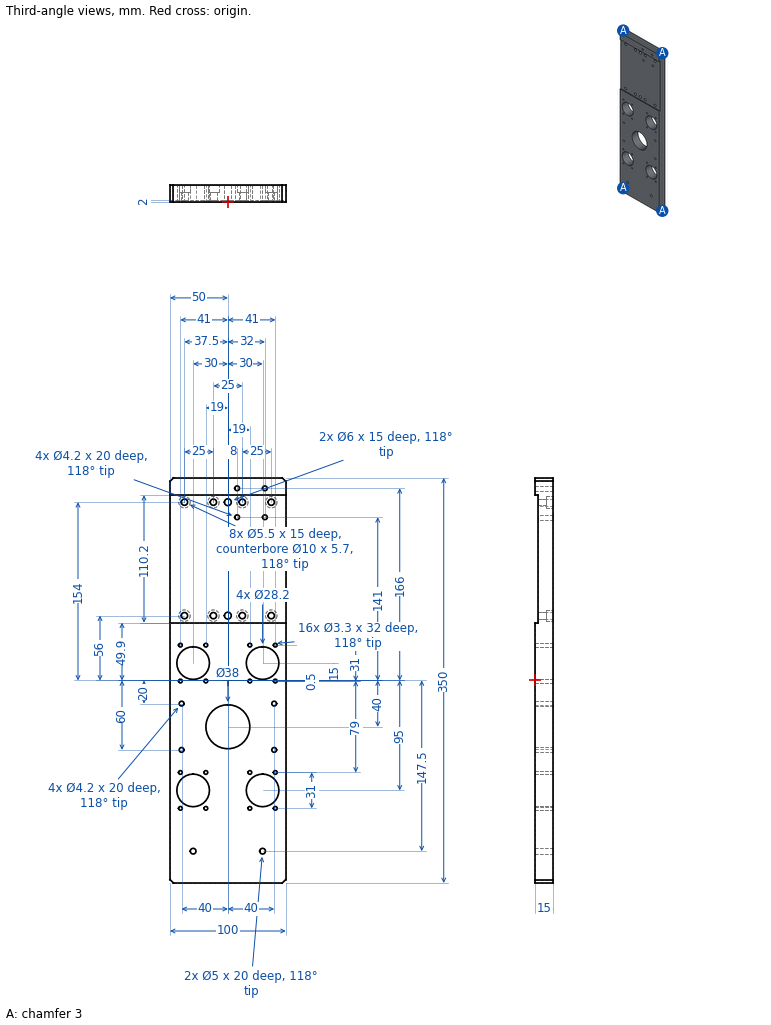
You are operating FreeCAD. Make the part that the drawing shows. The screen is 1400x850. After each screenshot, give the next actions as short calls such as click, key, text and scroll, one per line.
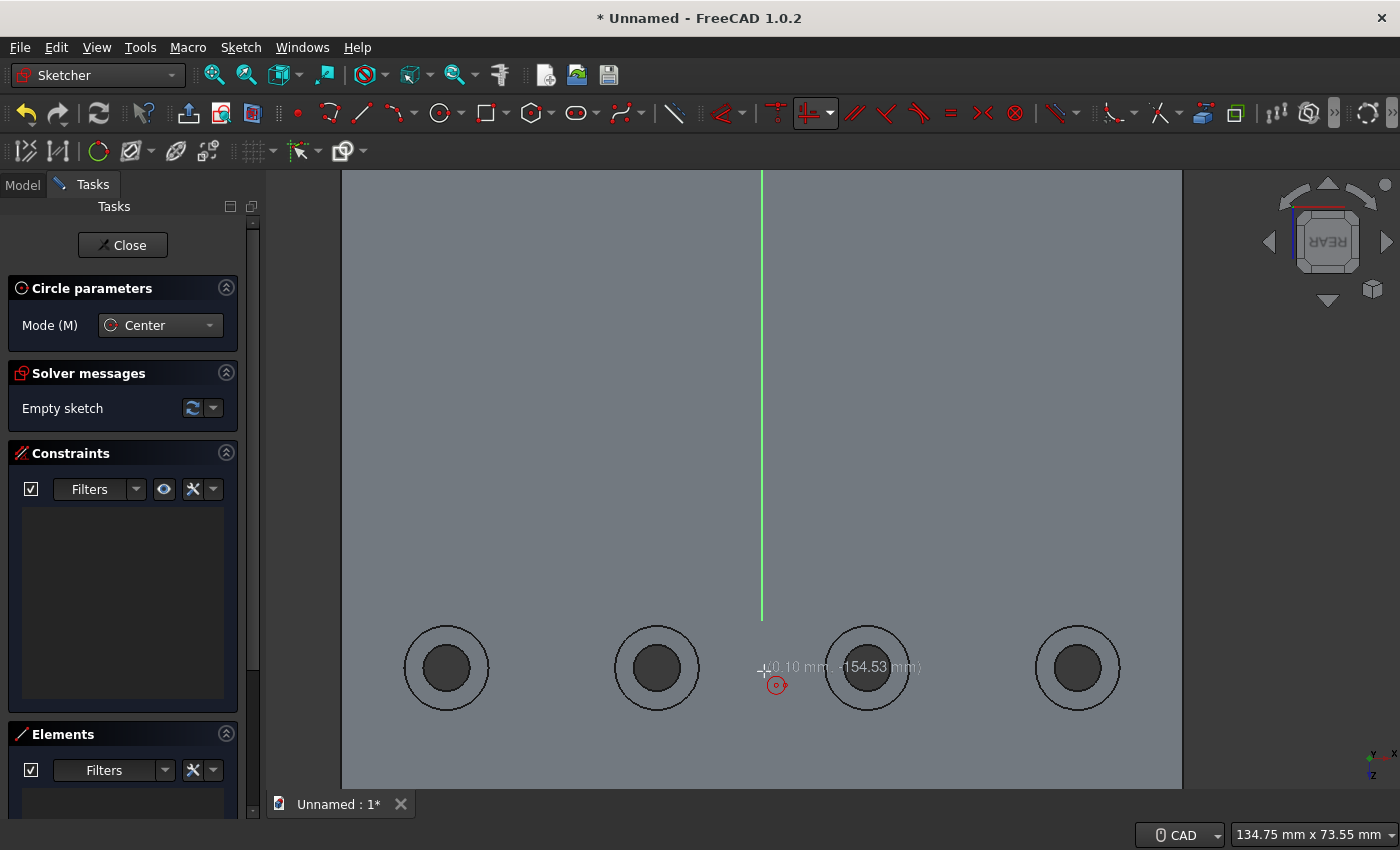
click(762, 668)
click(780, 650)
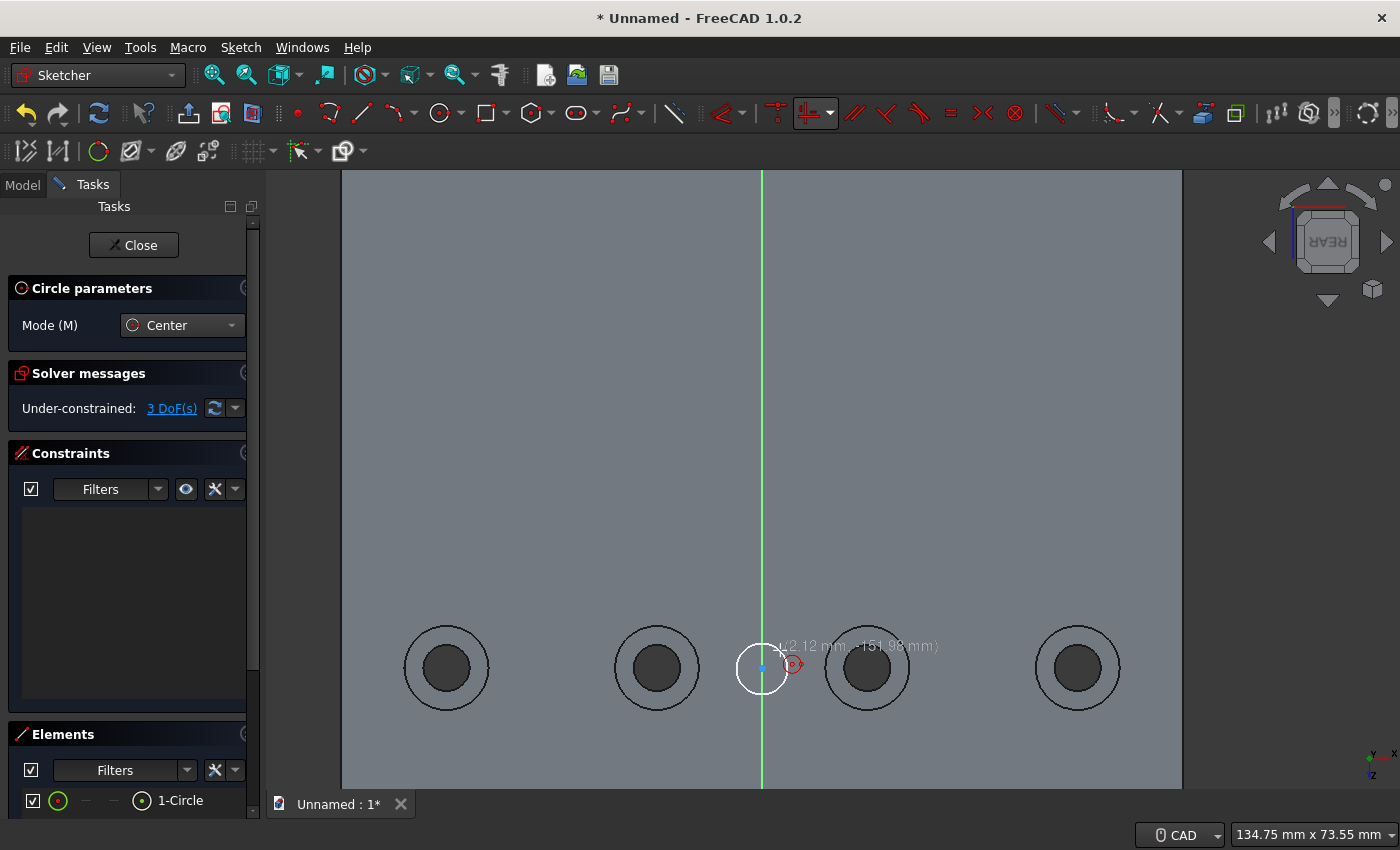
scroll(766, 672, down, 6)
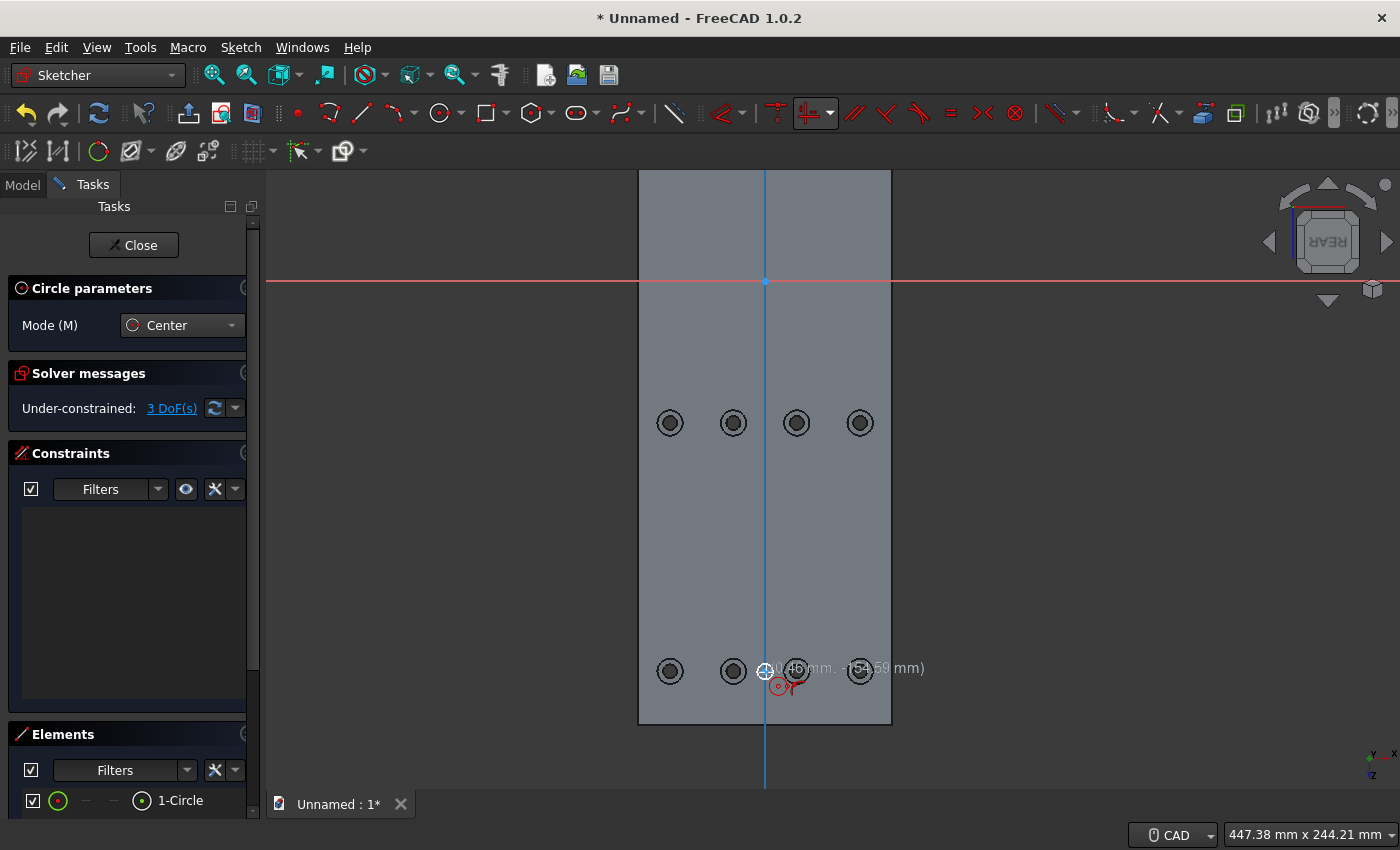
scroll(765, 423, up, 6)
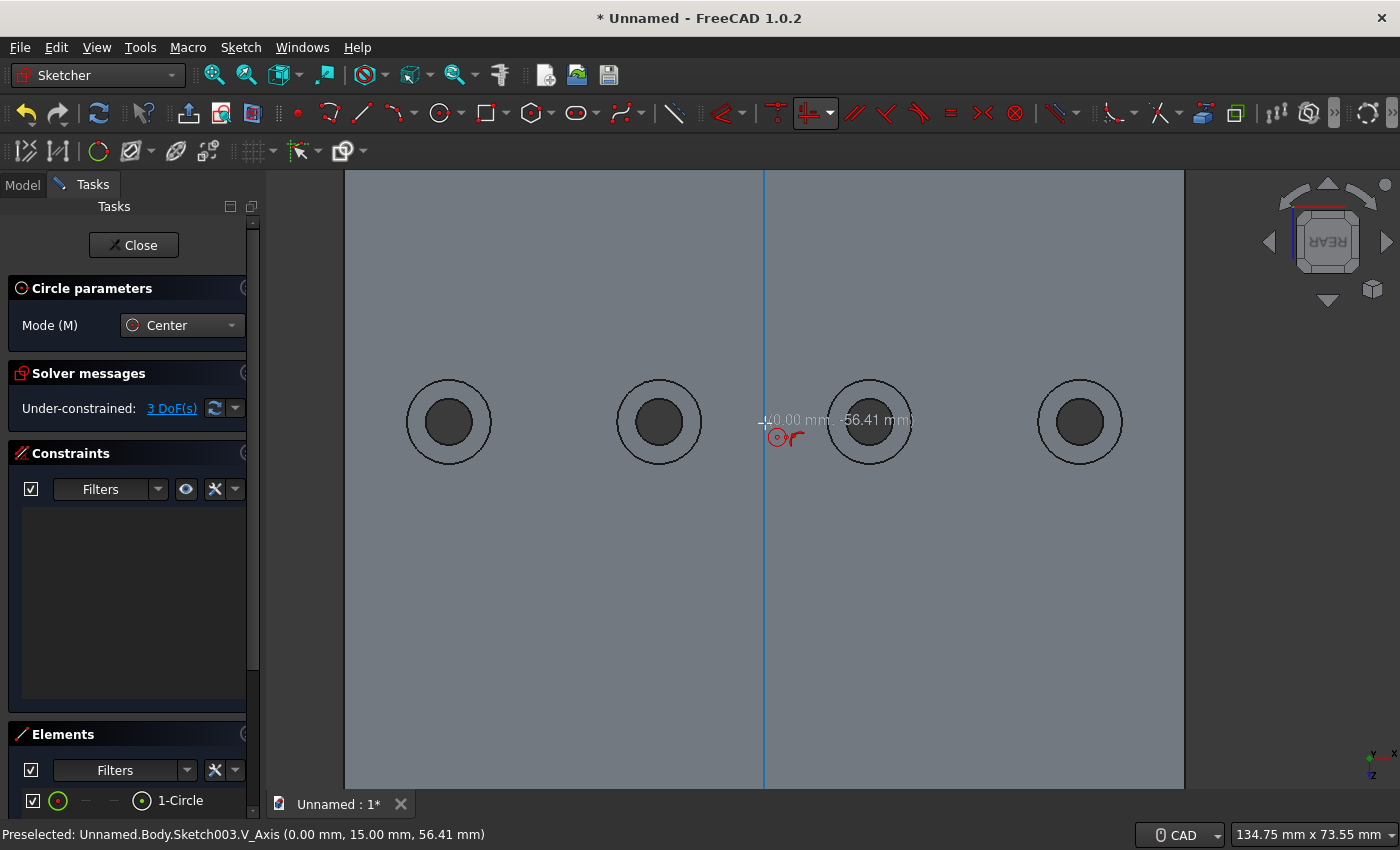
click(764, 422)
click(782, 404)
key(Escape)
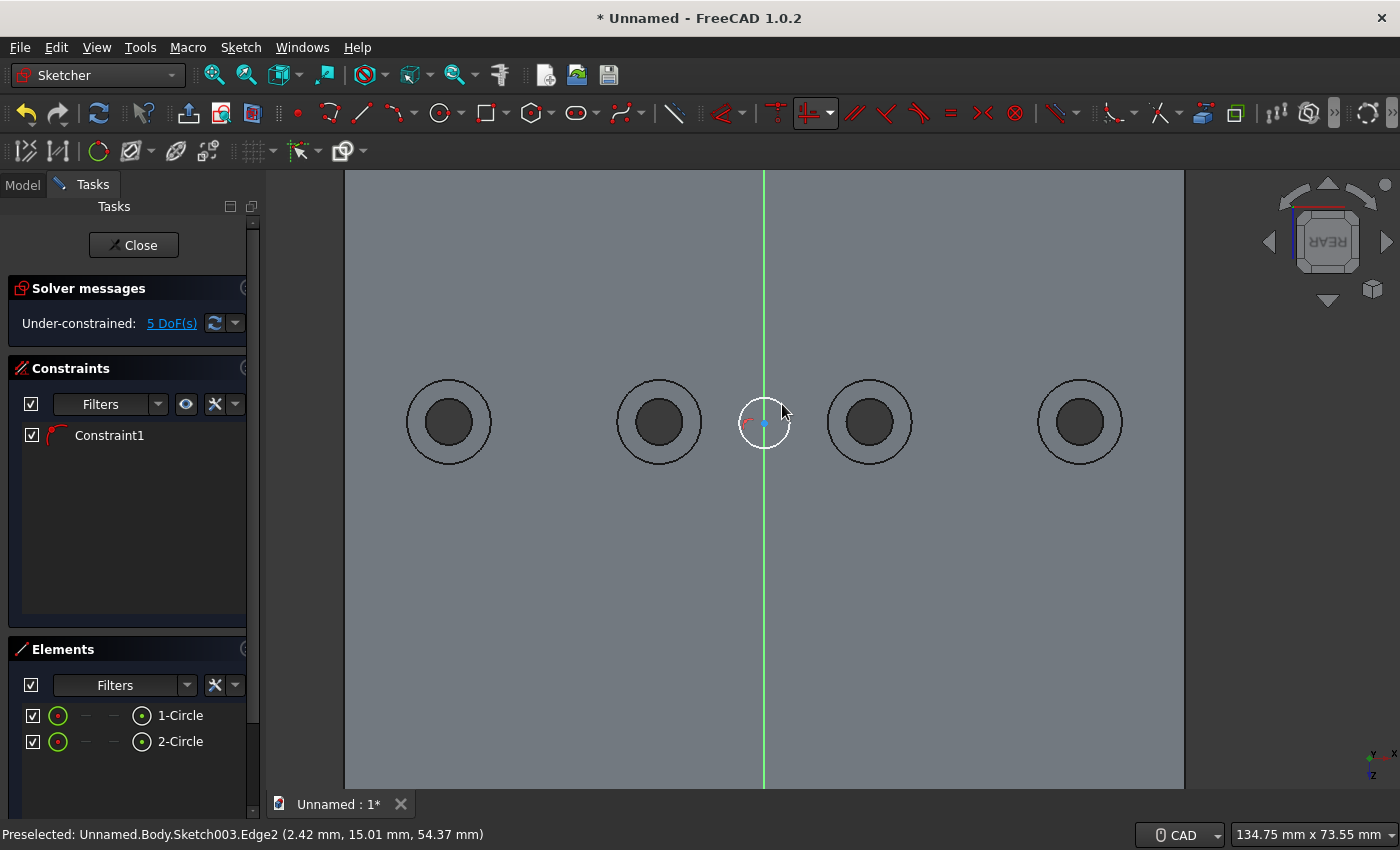
scroll(765, 423, down, 6)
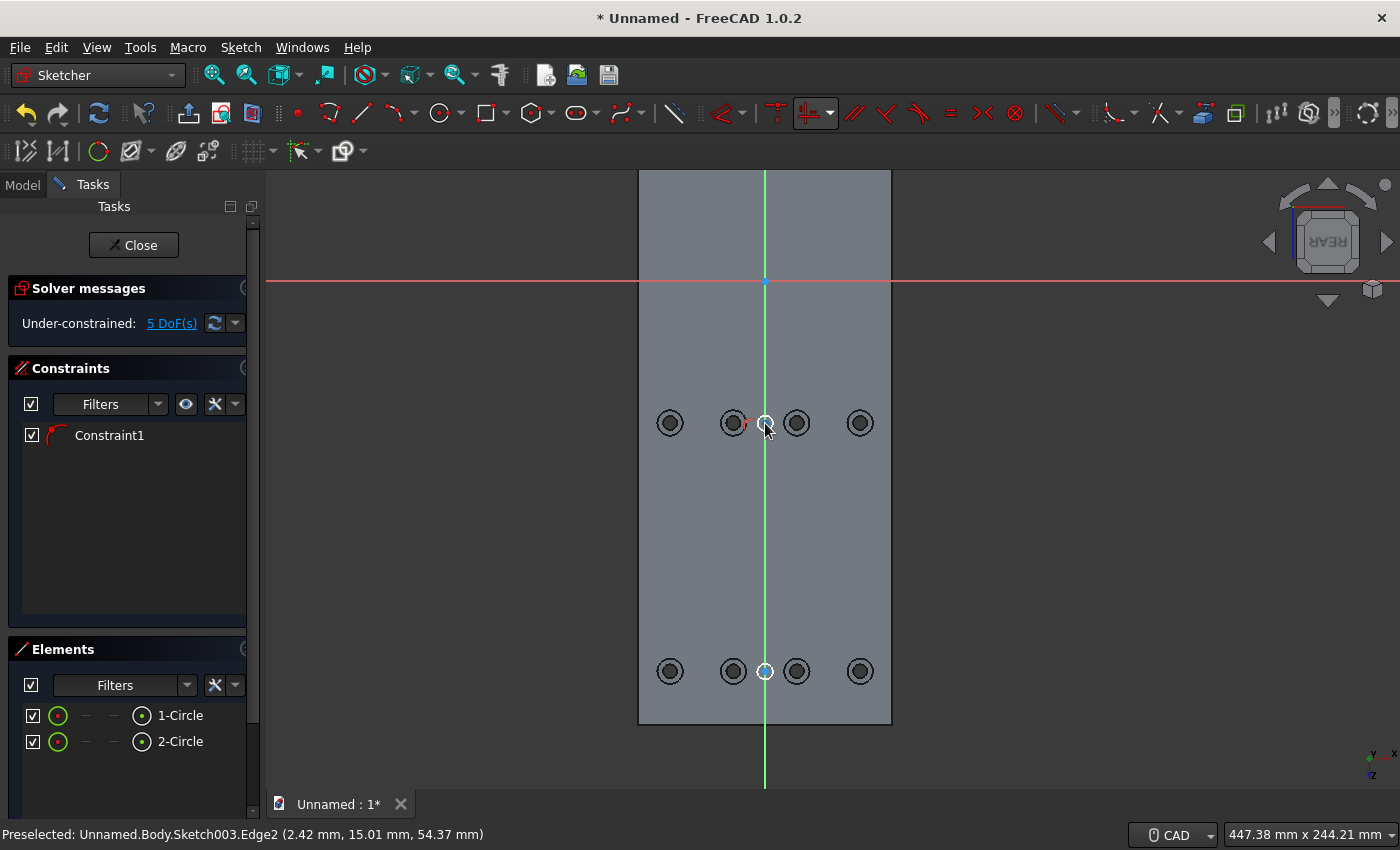
scroll(771, 666, up, 5)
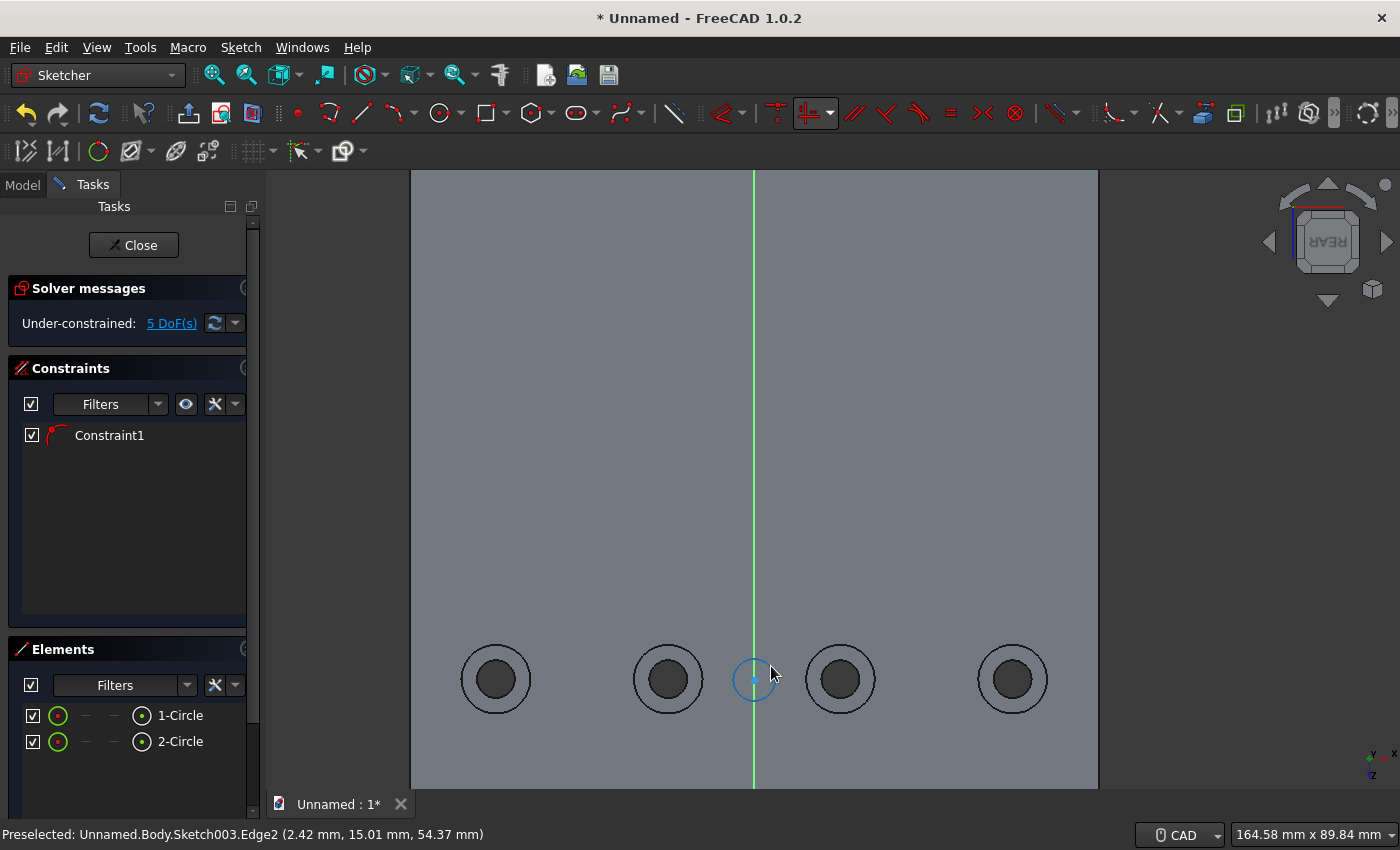
click(769, 665)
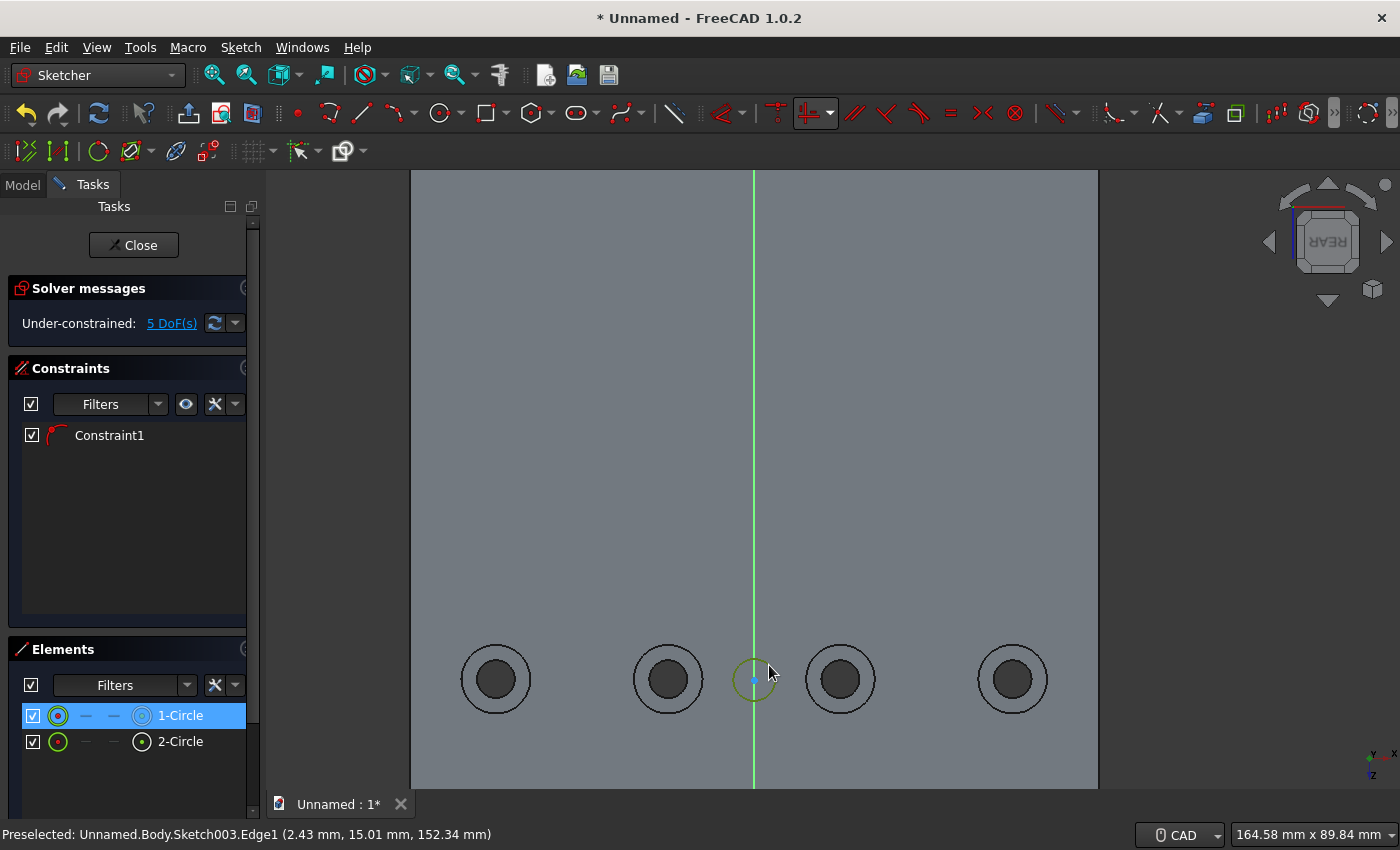
scroll(770, 666, down, 5)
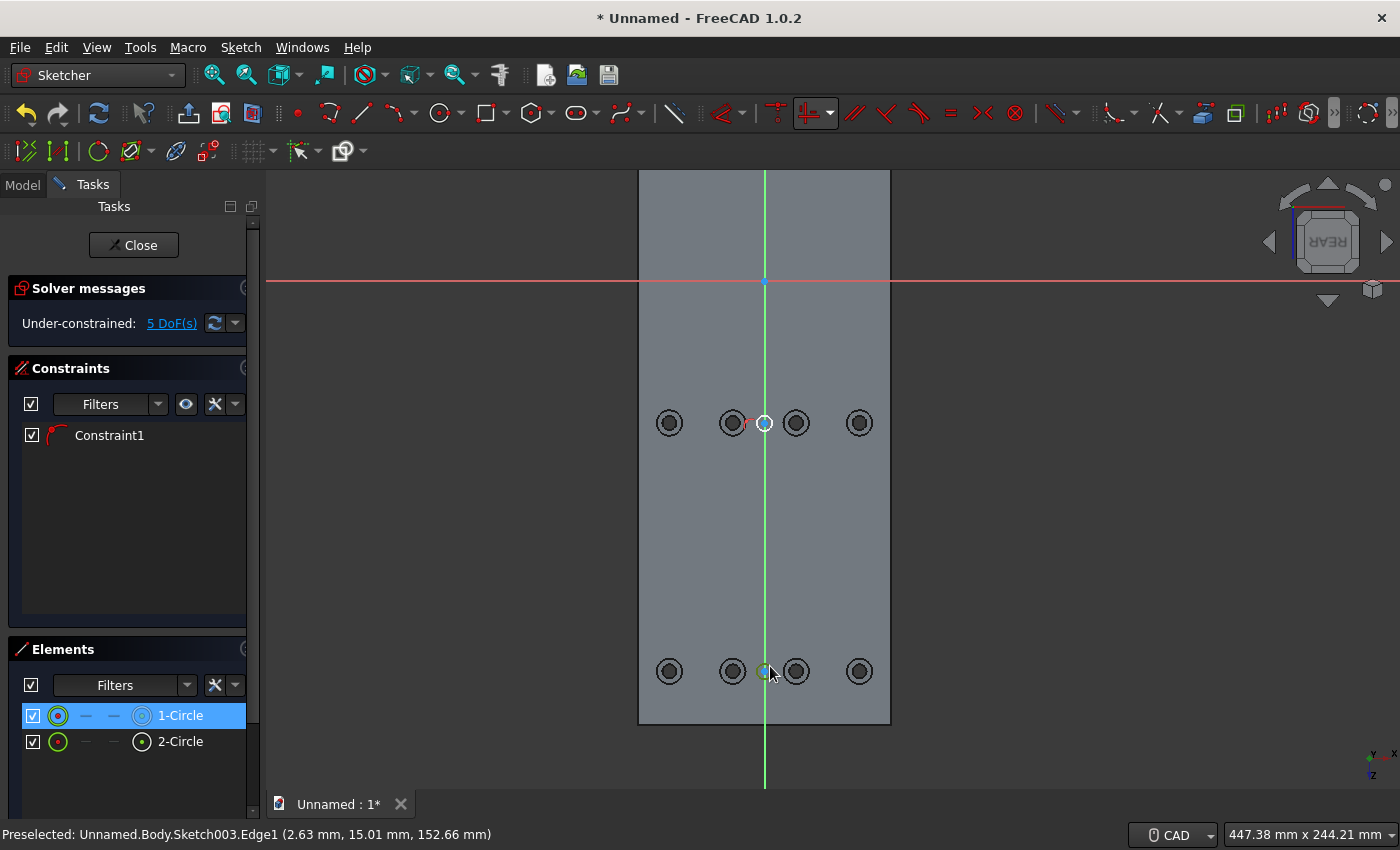
scroll(770, 418, up, 5)